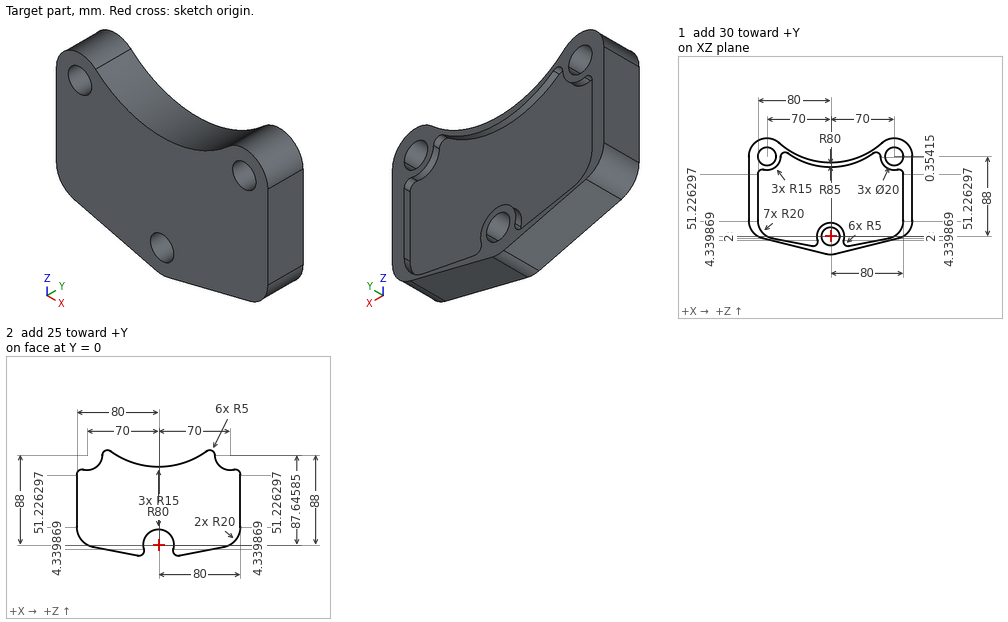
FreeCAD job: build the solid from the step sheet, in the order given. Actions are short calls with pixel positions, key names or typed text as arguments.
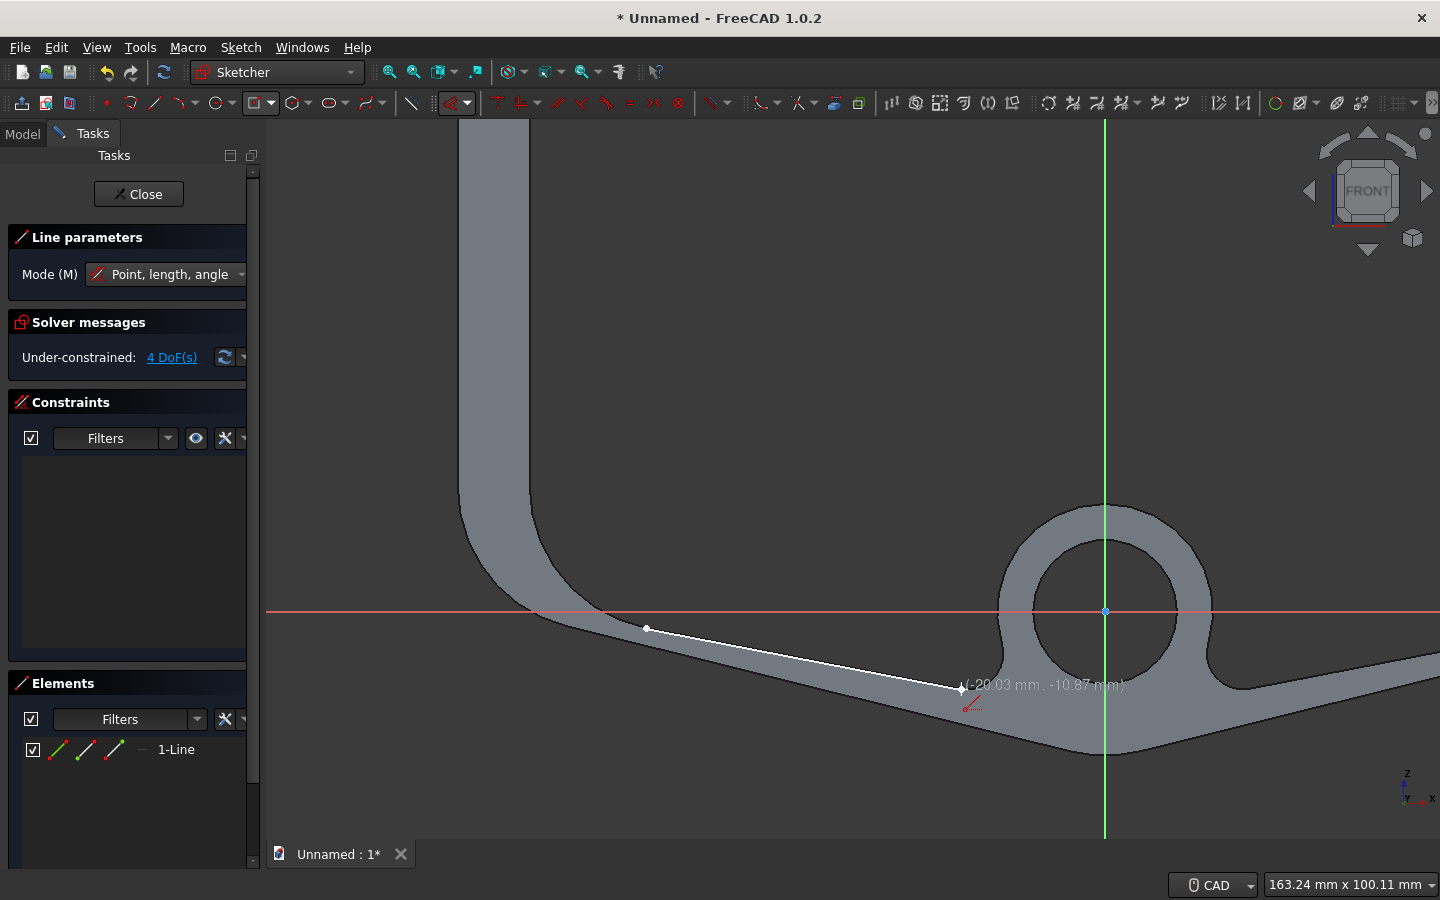
click(1250, 689)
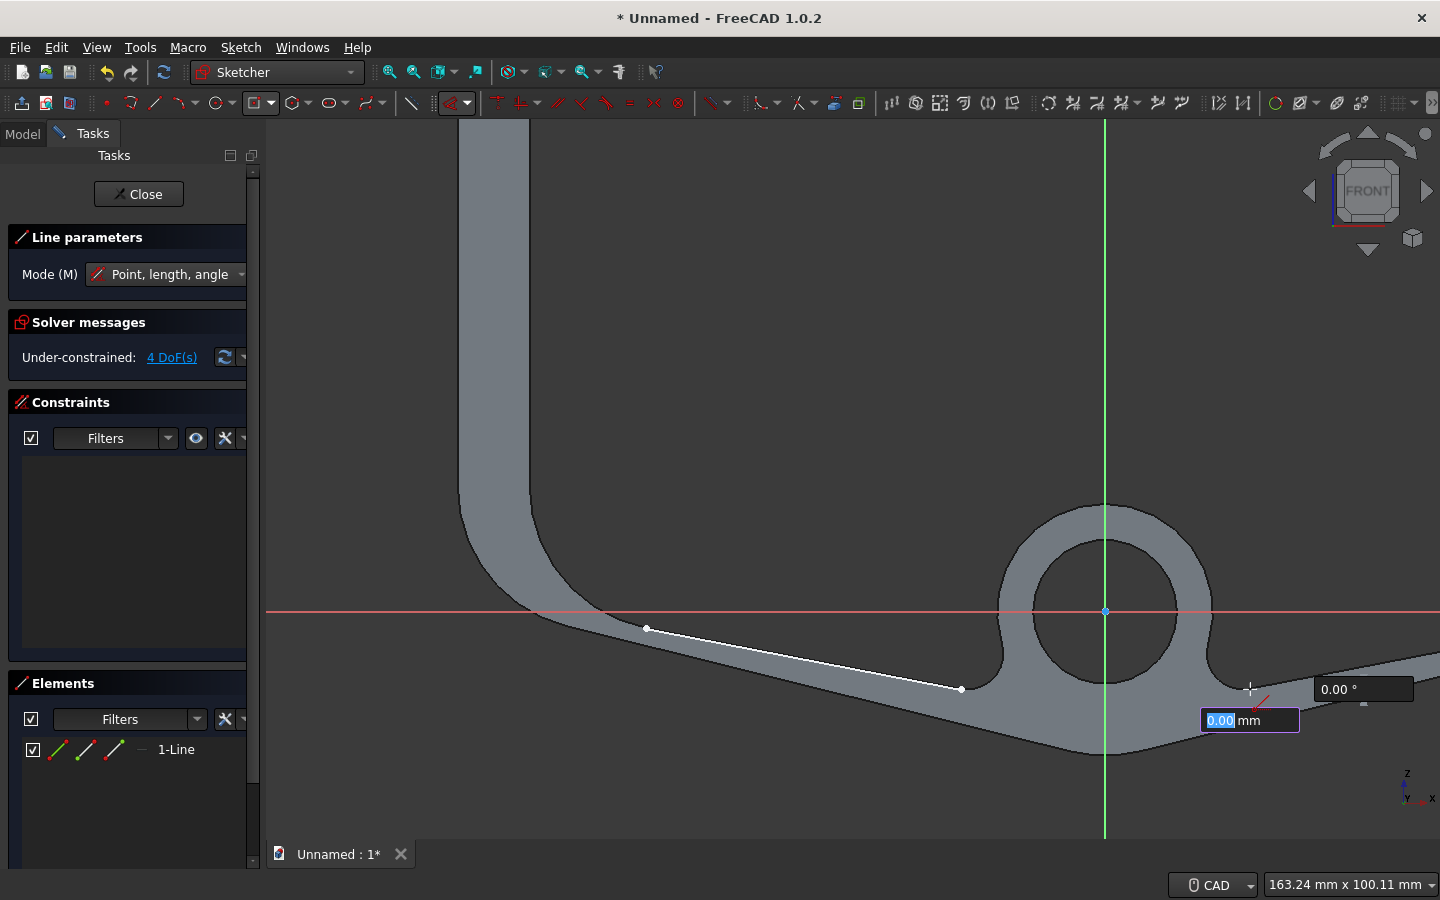
scroll(395, 673, down, 3)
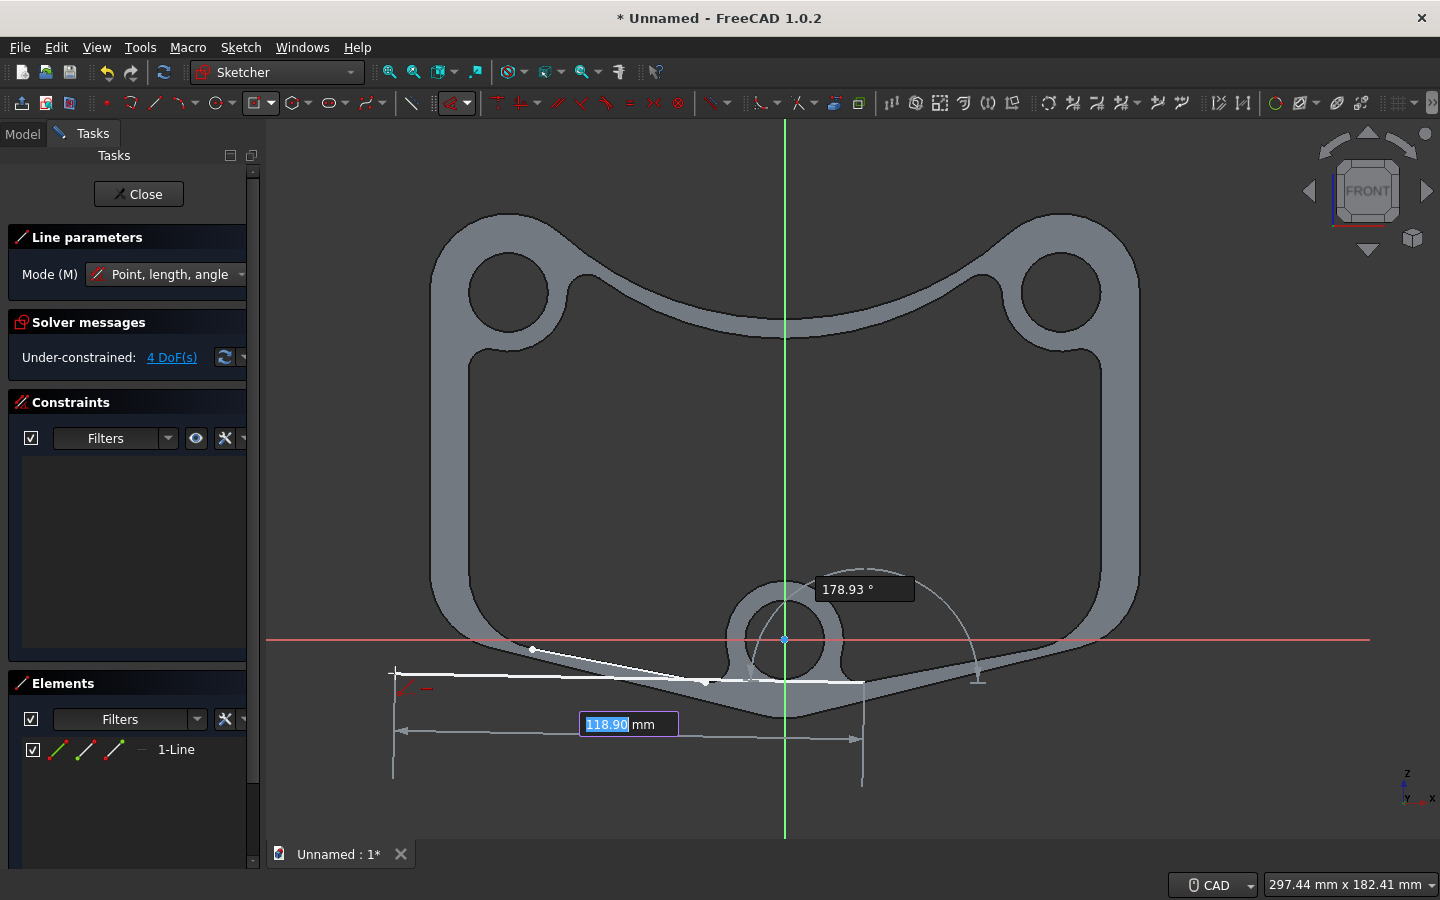
scroll(1037, 649, up, 3)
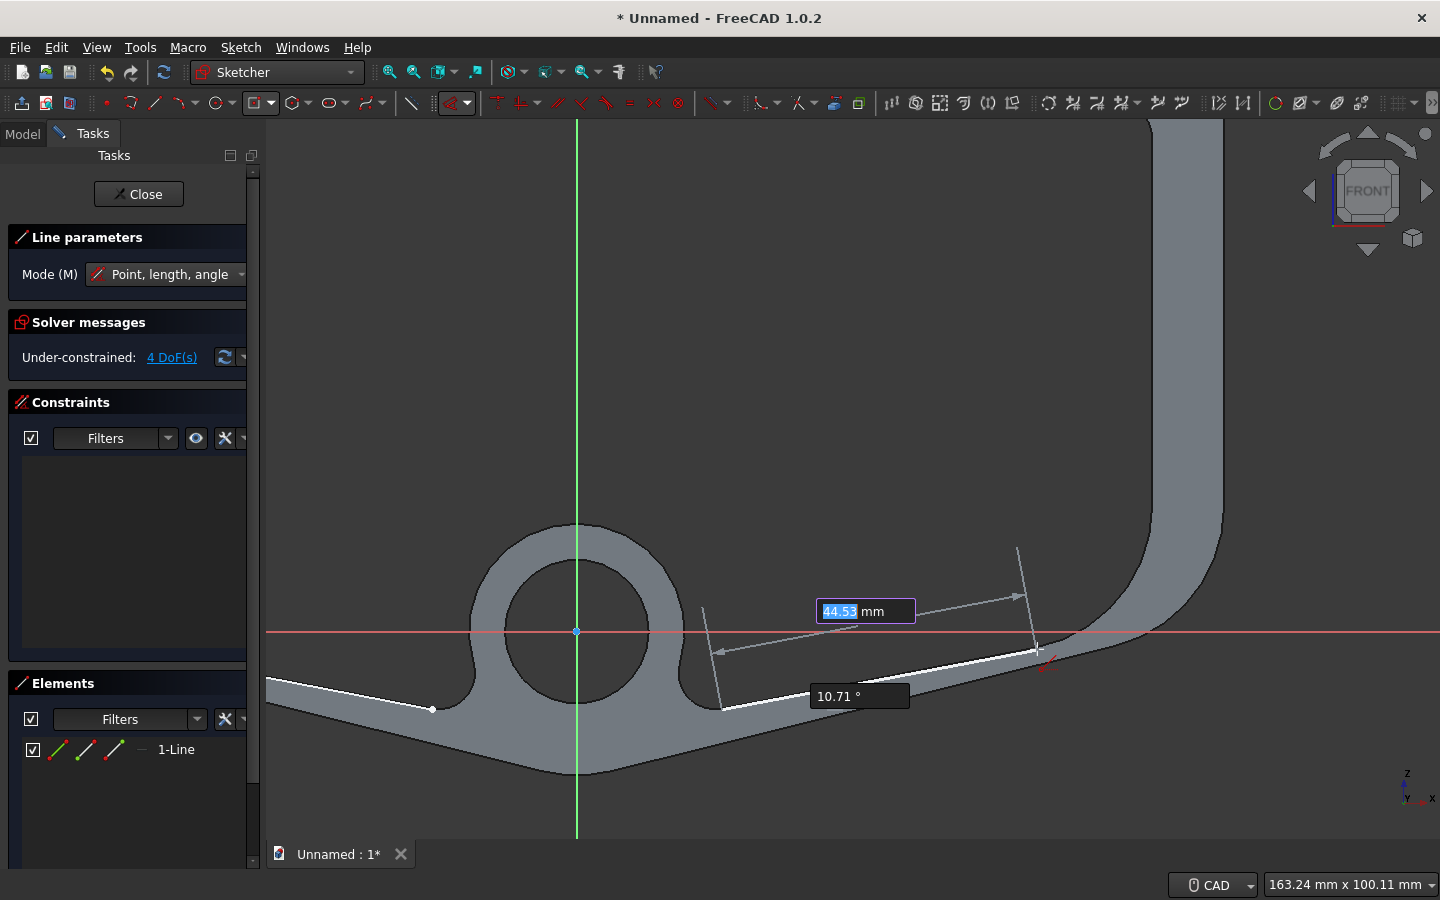
click(1036, 648)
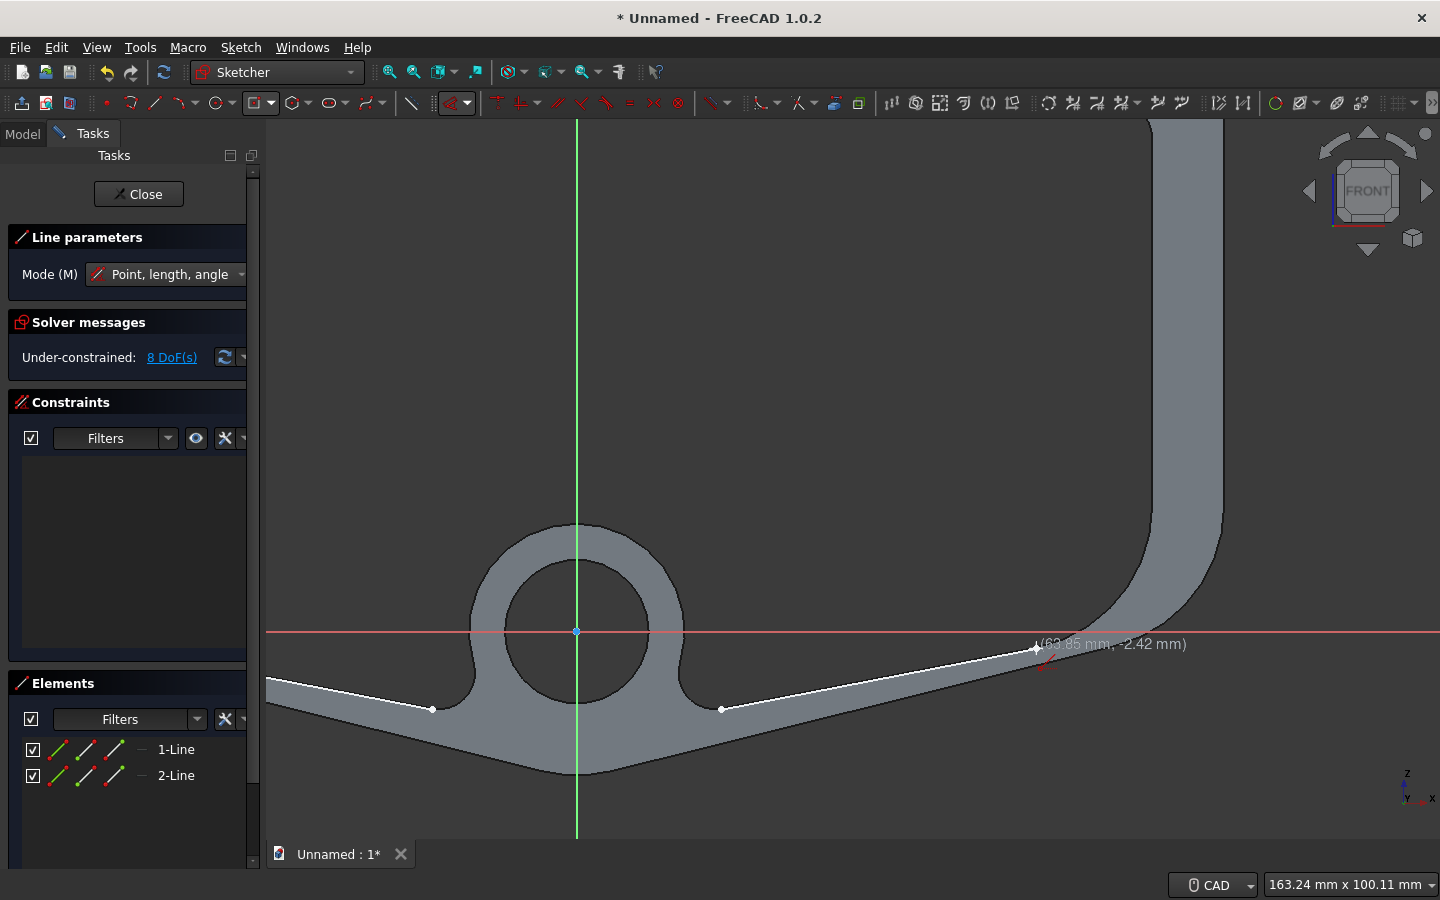
click(1152, 506)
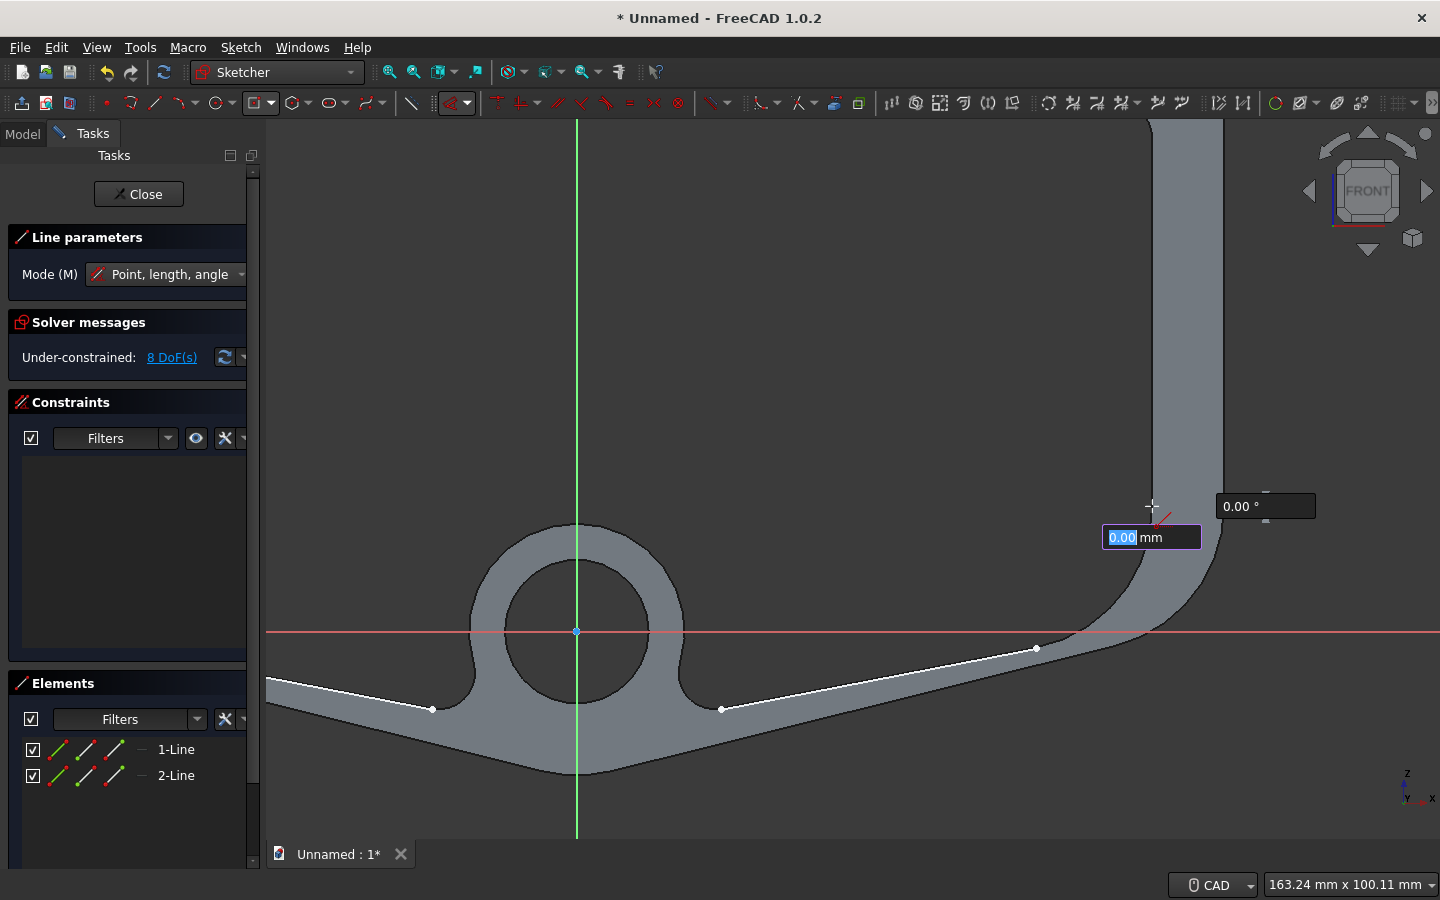
scroll(1037, 649, down, 3)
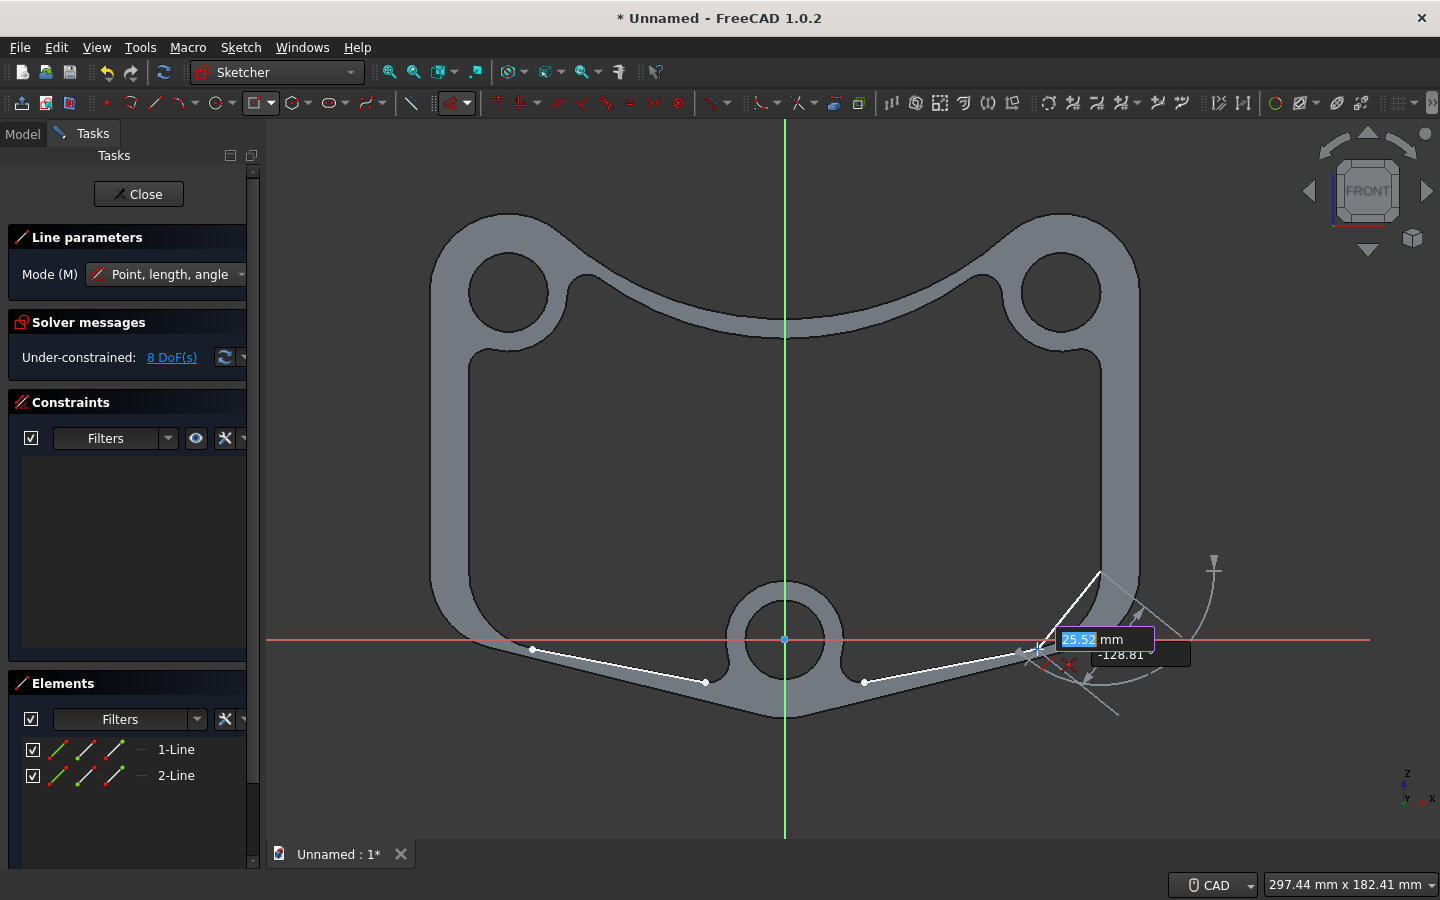
click(1100, 369)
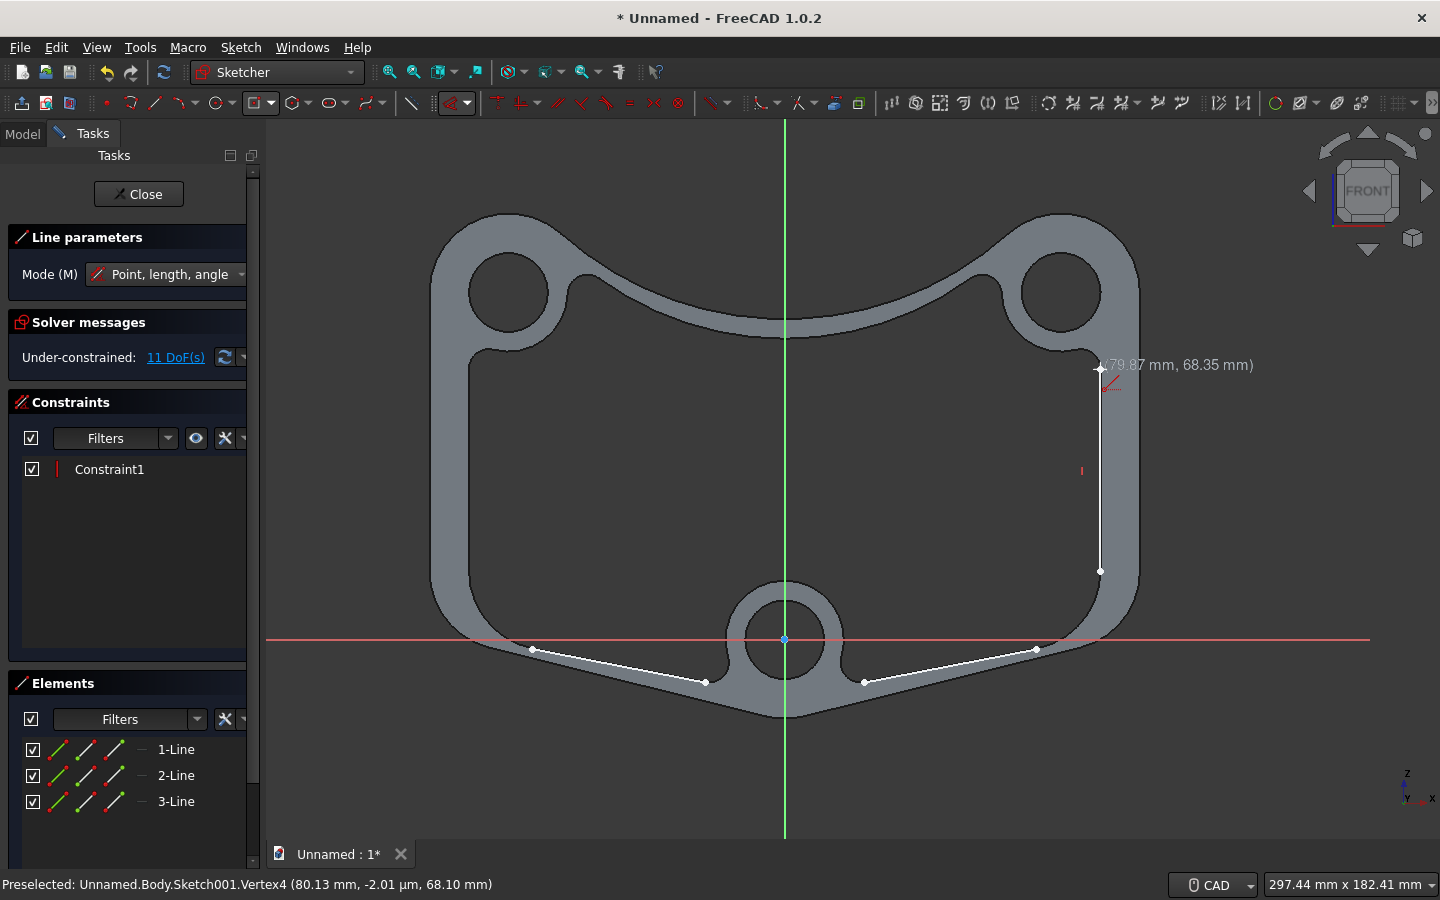
click(469, 369)
click(469, 571)